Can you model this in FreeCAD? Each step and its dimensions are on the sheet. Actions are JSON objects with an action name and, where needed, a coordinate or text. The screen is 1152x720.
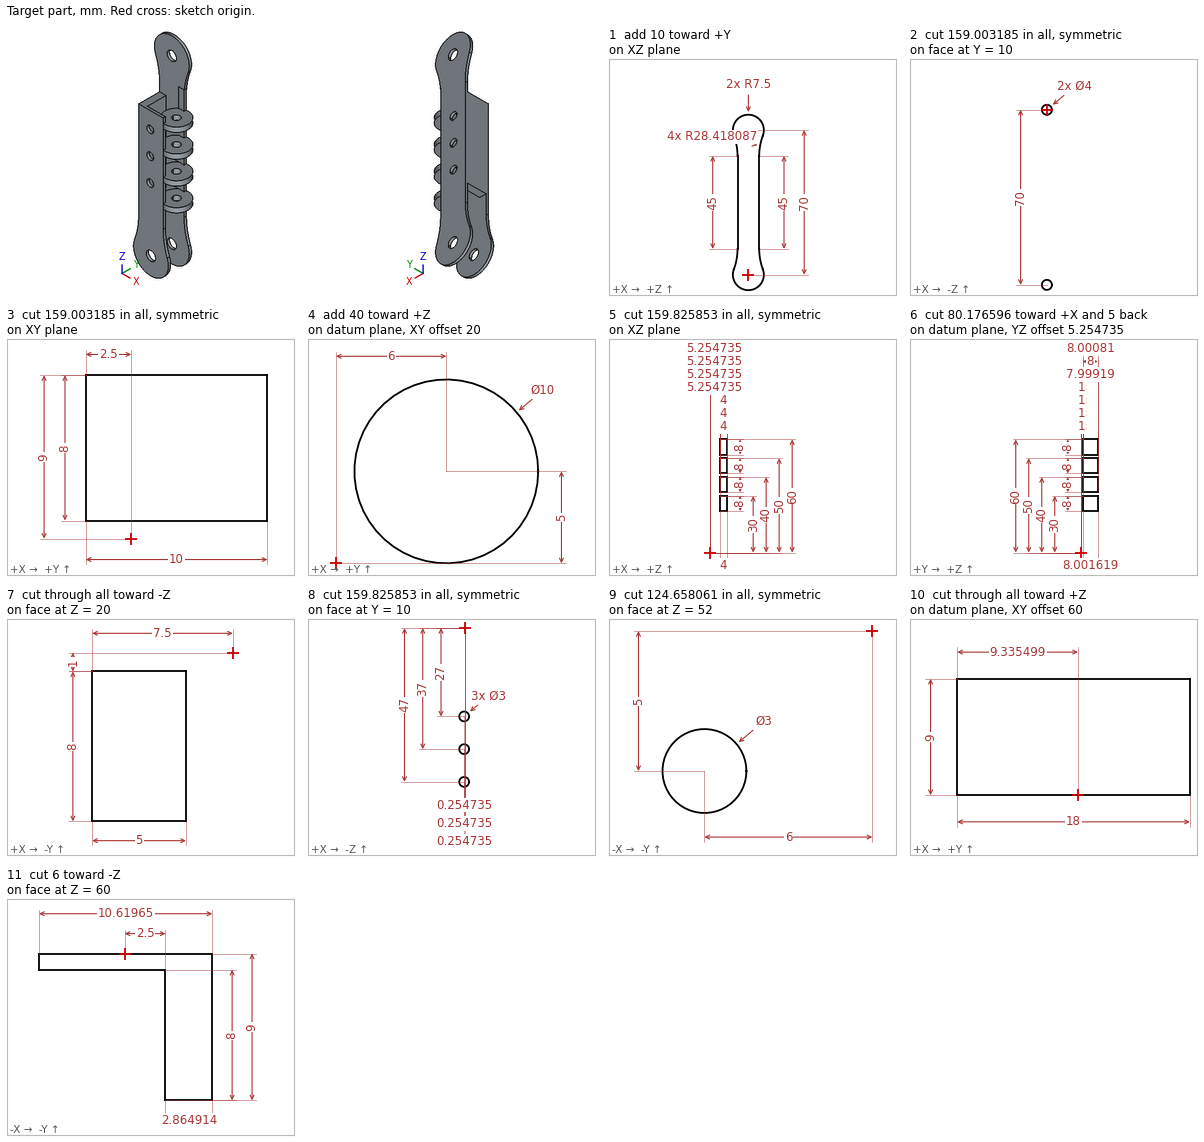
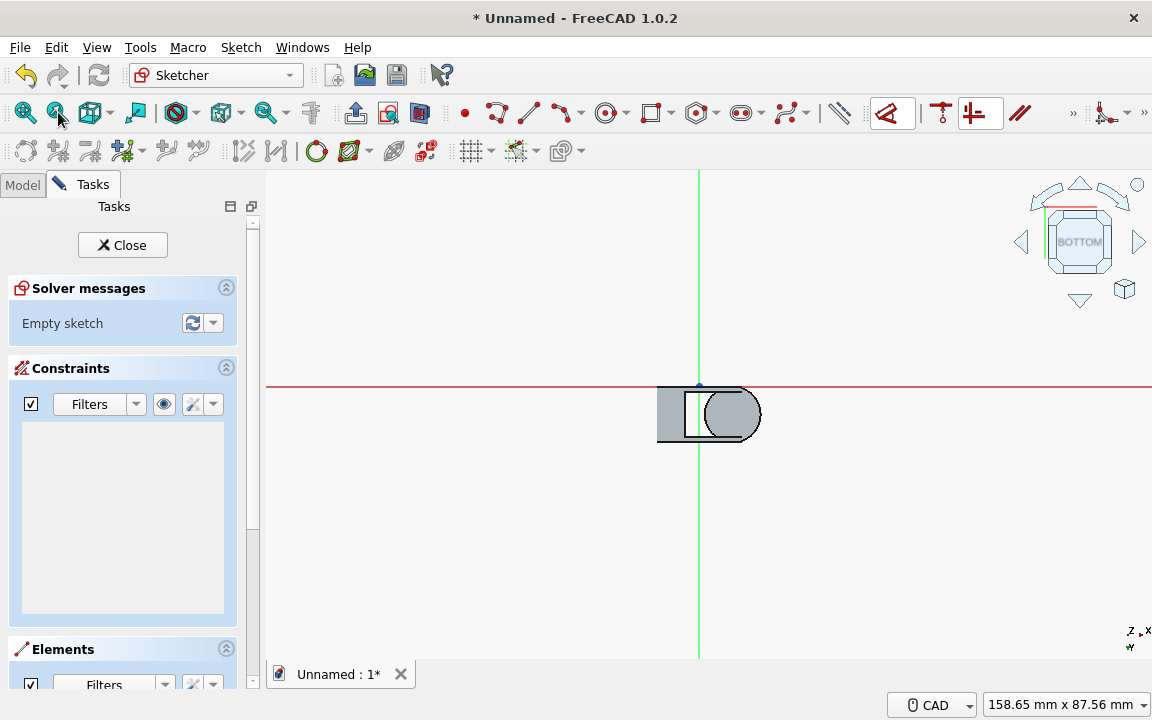
{"action": "left_click", "coordinate": [420, 114]}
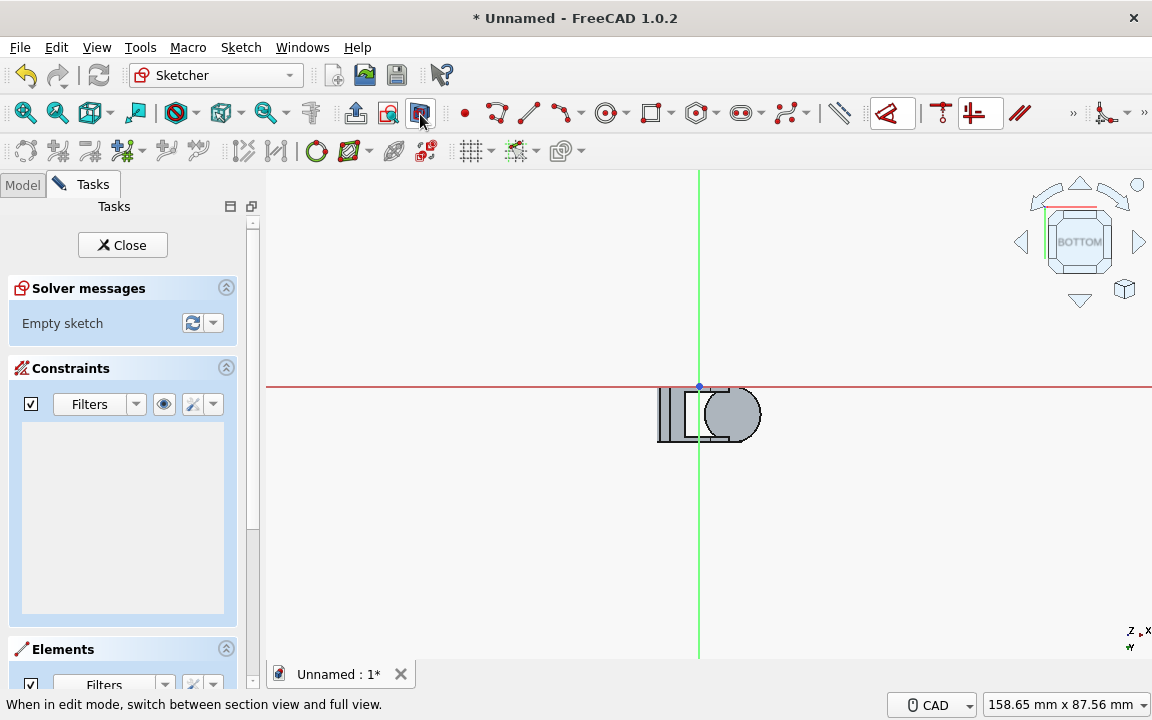
{"action": "scroll", "coordinate": [686, 411], "scroll_direction": "up", "scroll_amount": 9}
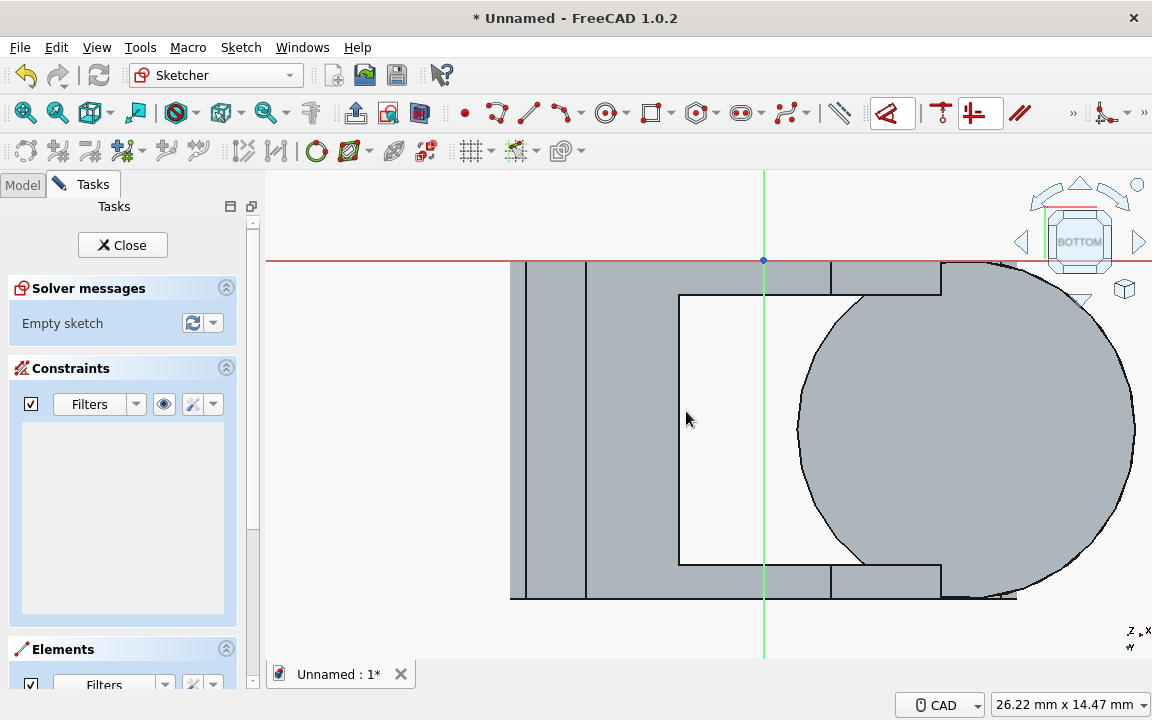
{"action": "key", "text": "g r"}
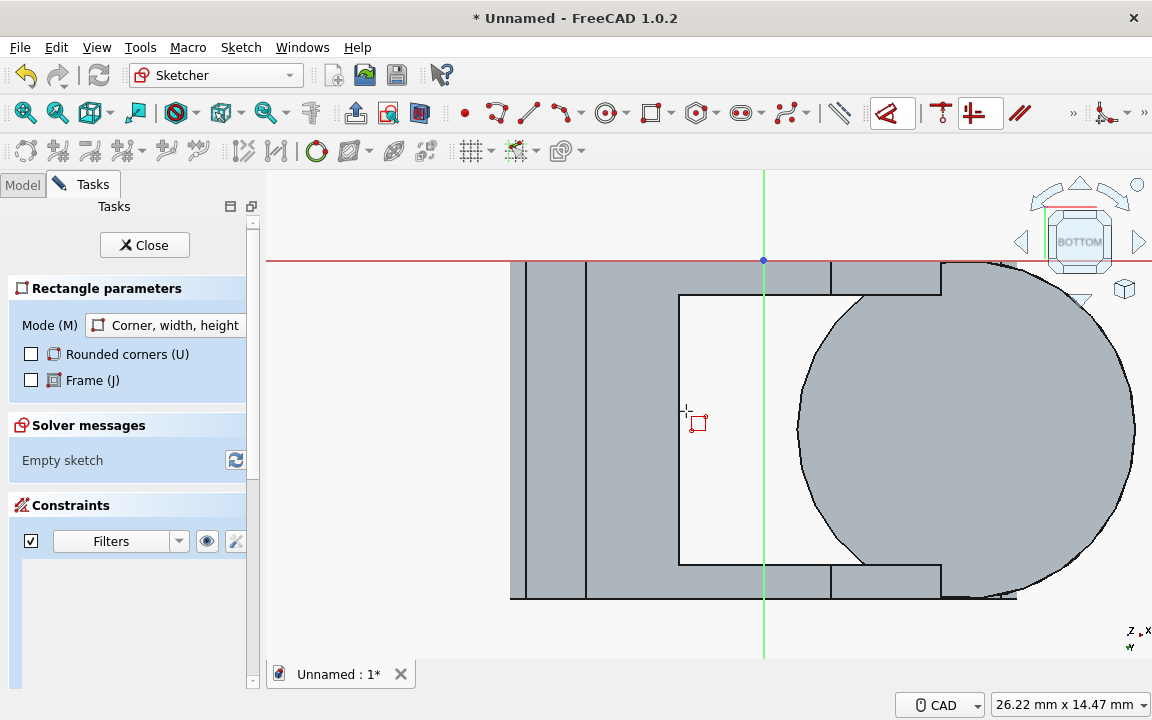
{"action": "left_click", "coordinate": [510, 295]}
{"action": "left_click", "coordinate": [679, 565]}
{"action": "key", "text": "Escape"}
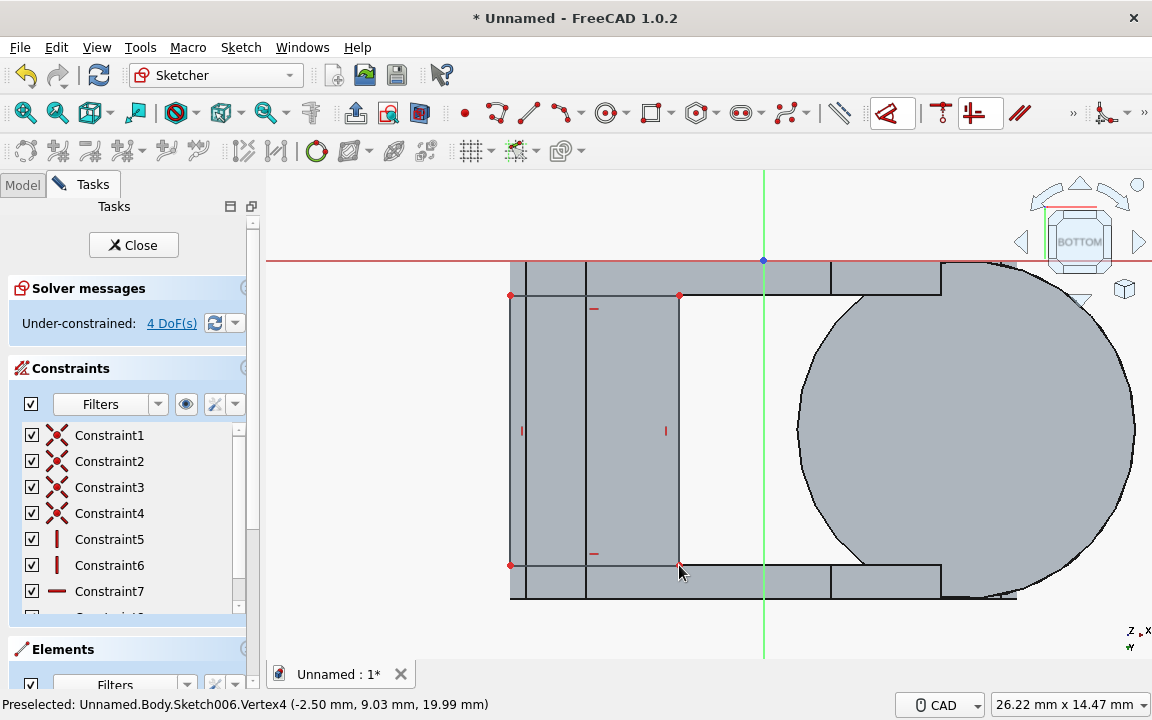
{"action": "left_click", "coordinate": [510, 377]}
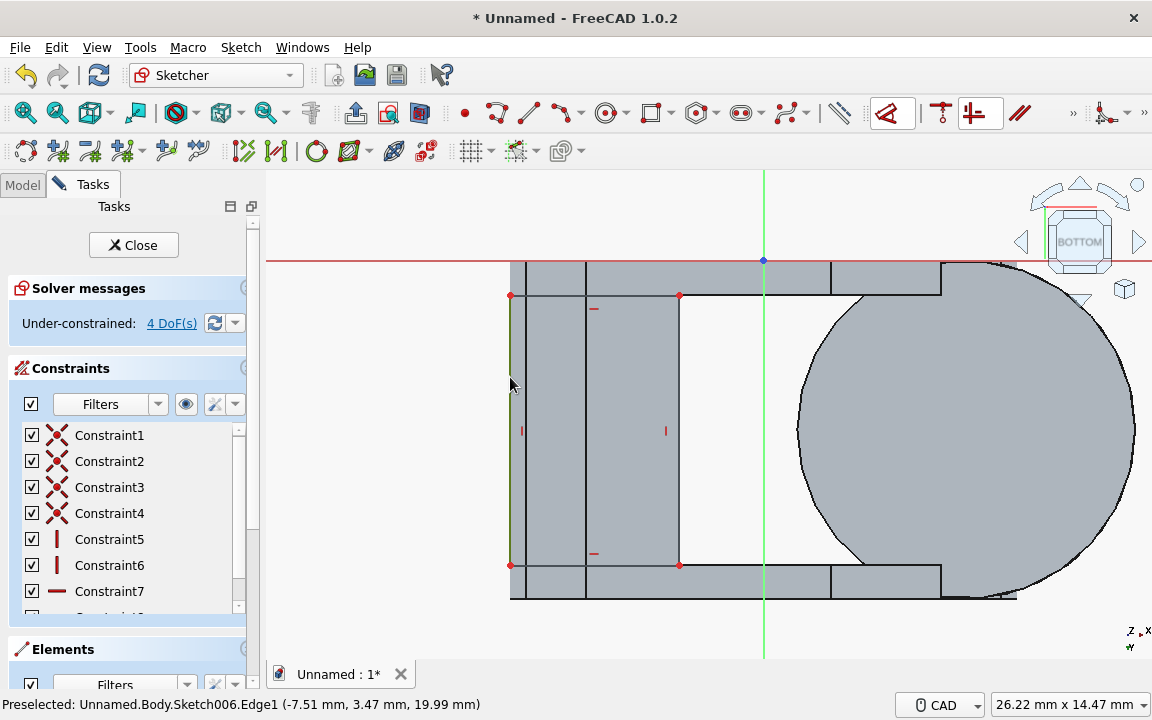
{"action": "left_click", "coordinate": [910, 114]}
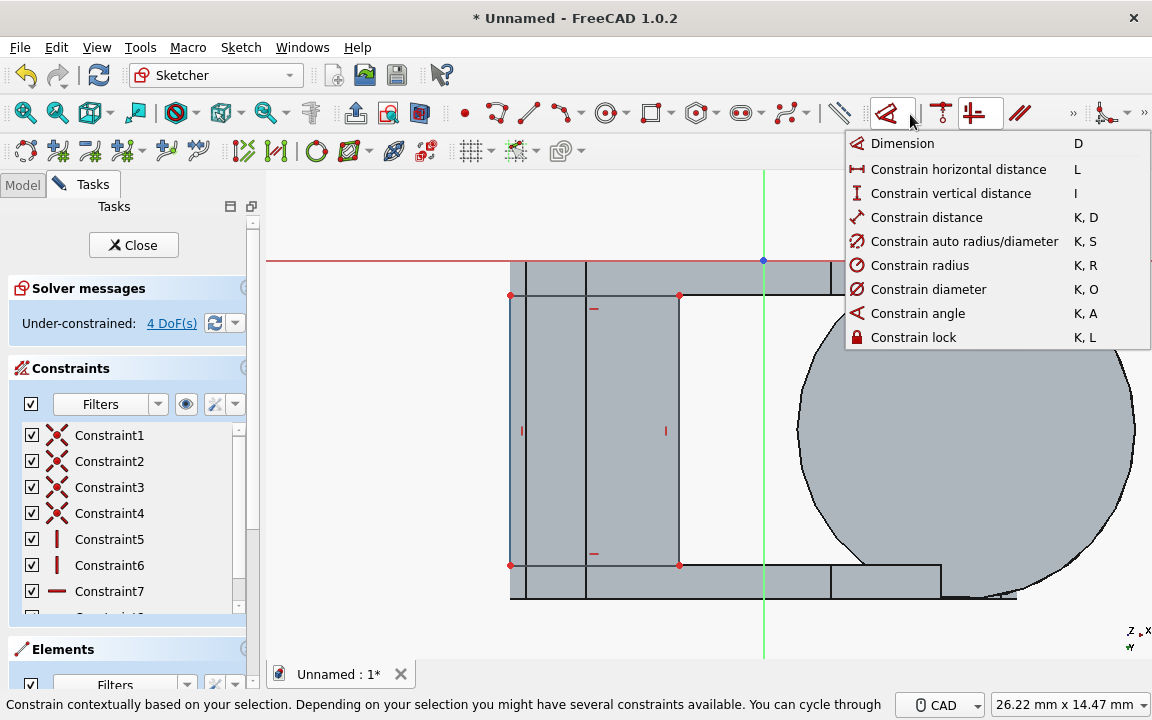
{"action": "left_click", "coordinate": [998, 193]}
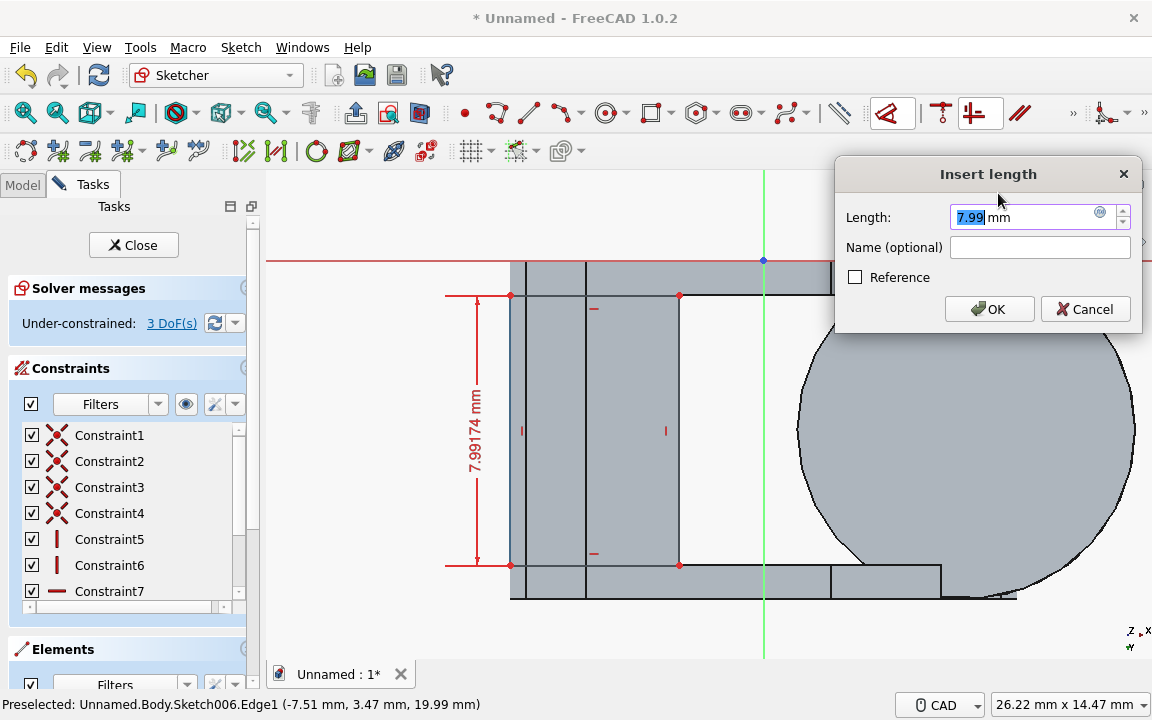
{"action": "type", "text": "8"}
{"action": "key", "text": "Return"}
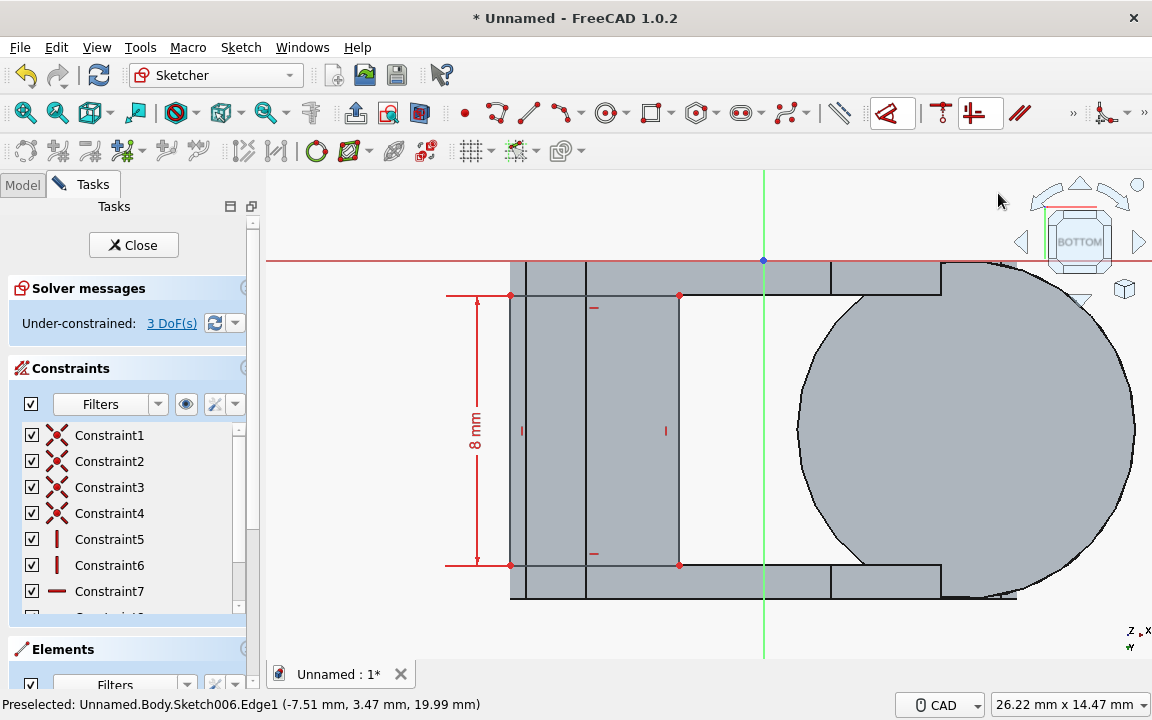
{"action": "left_click", "coordinate": [561, 566]}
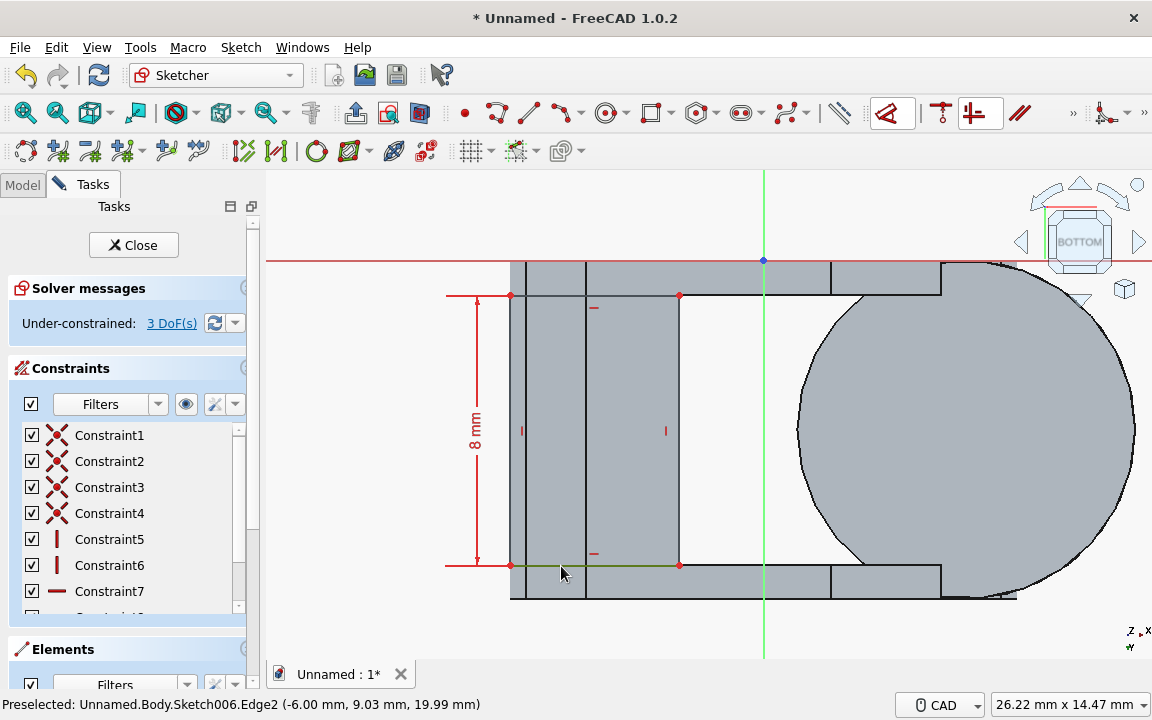
{"action": "key", "text": "l"}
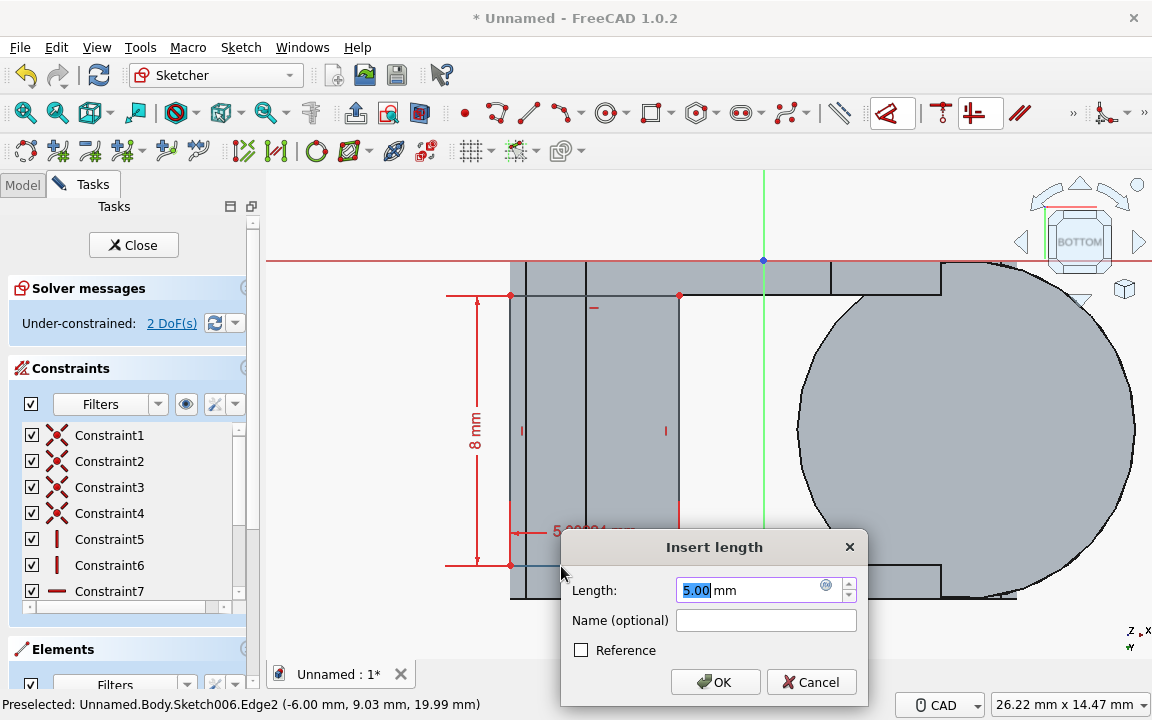
{"action": "type", "text": "5"}
{"action": "key", "text": "Return"}